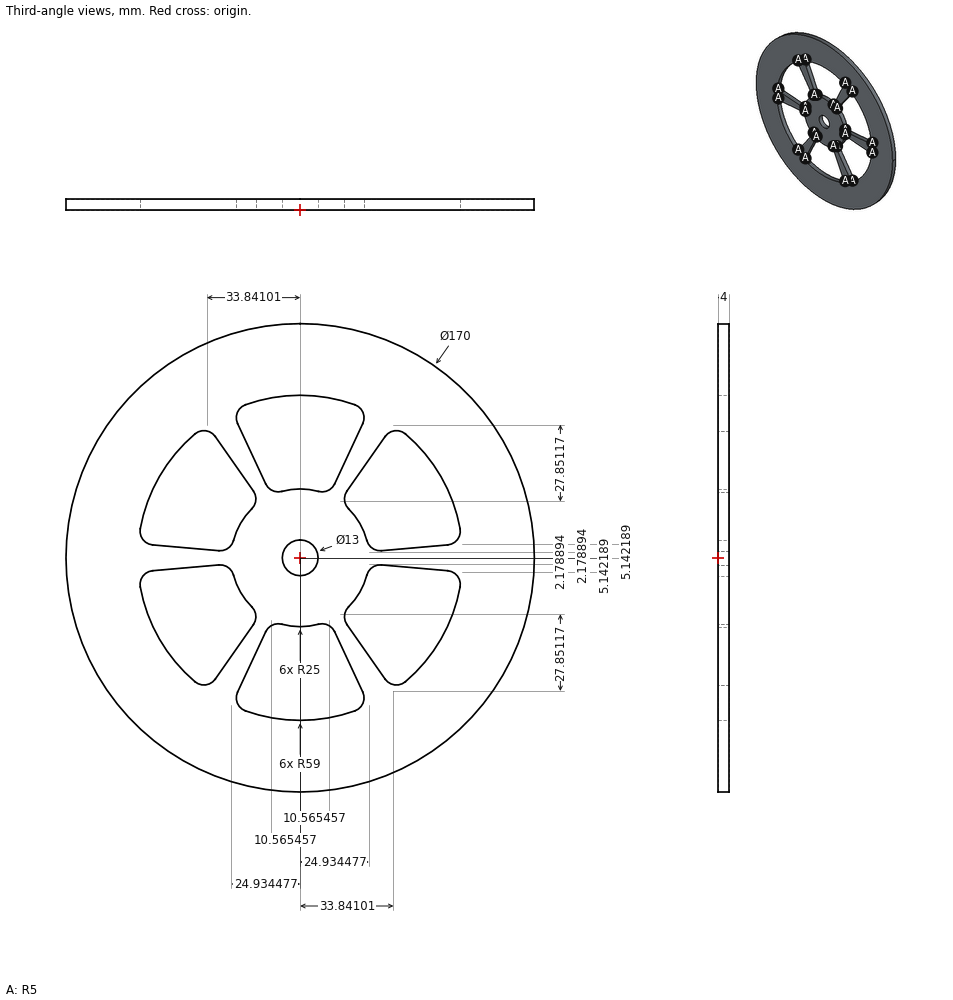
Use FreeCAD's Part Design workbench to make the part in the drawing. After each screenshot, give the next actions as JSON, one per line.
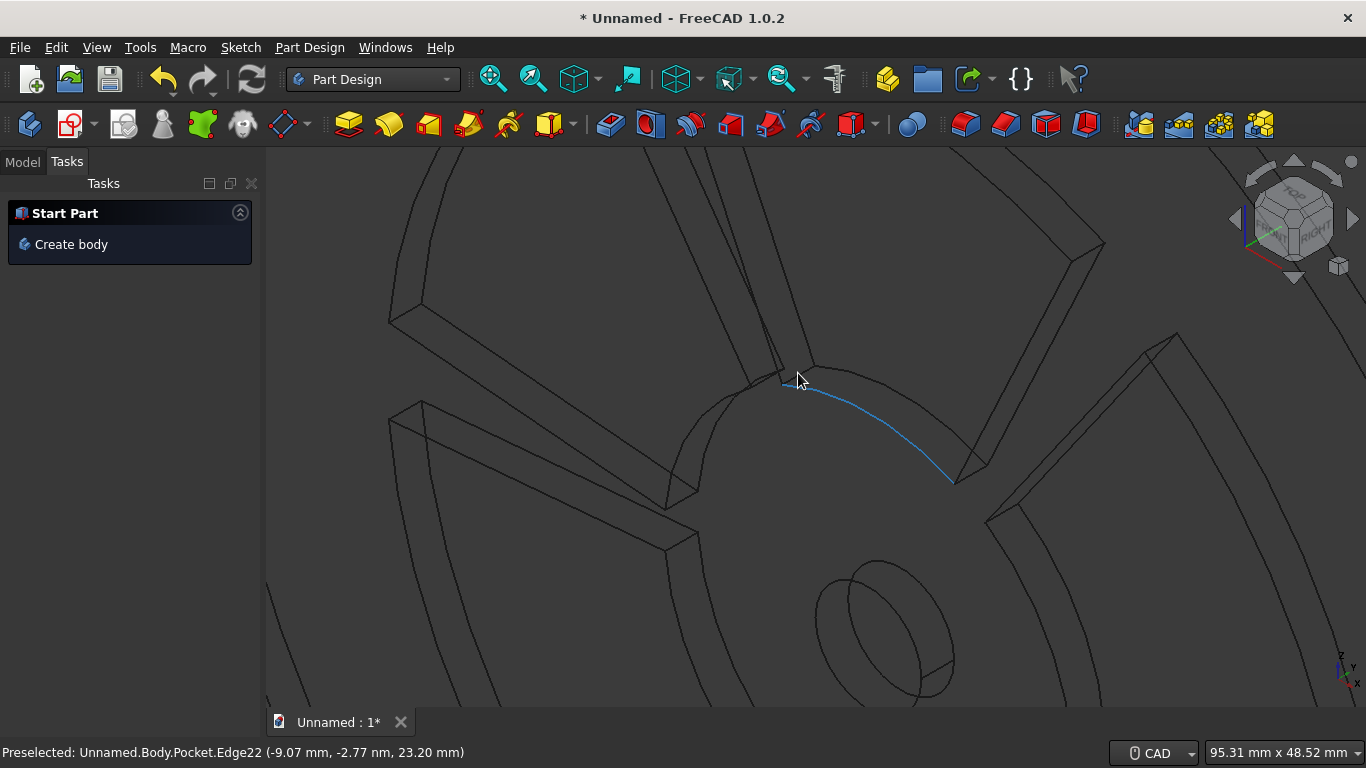
{"action": "left_click", "coordinate": [799, 374]}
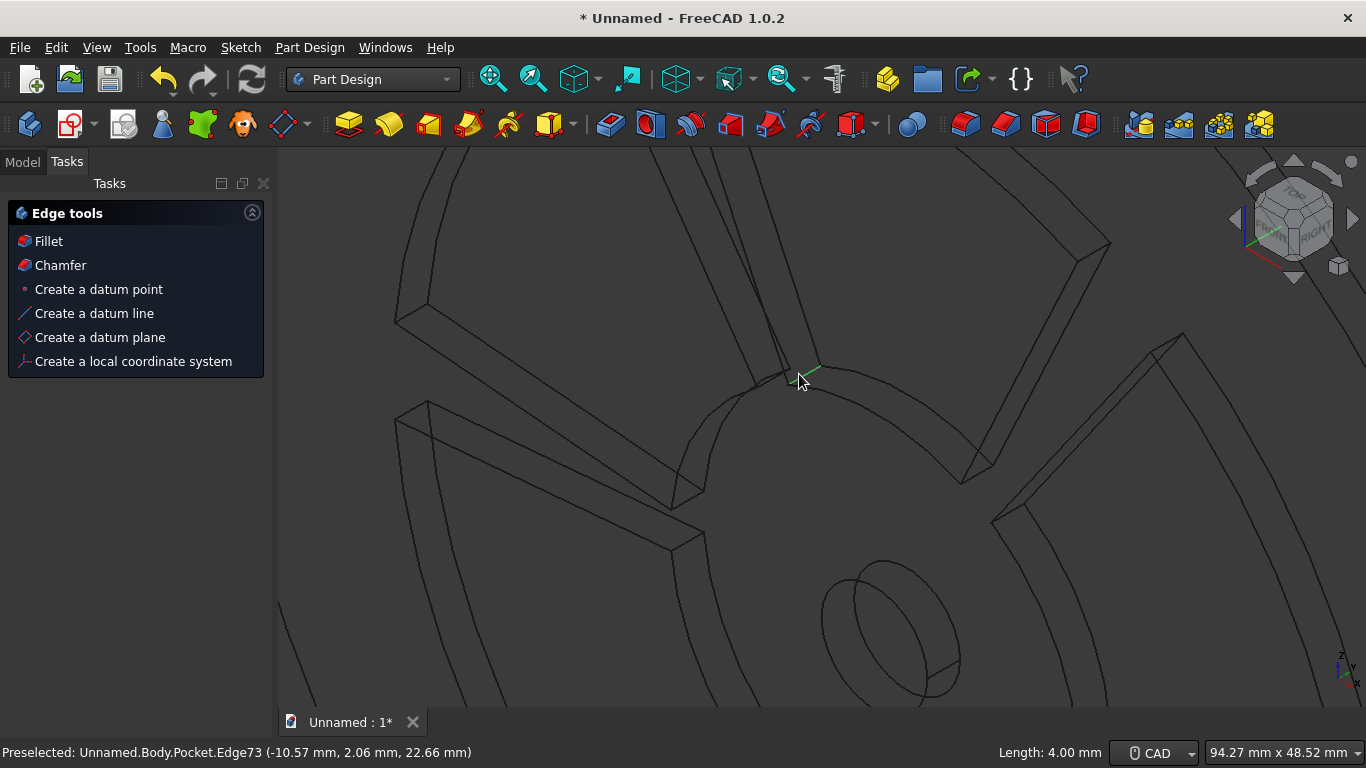
{"action": "left_click", "coordinate": [977, 474], "text": "ctrl"}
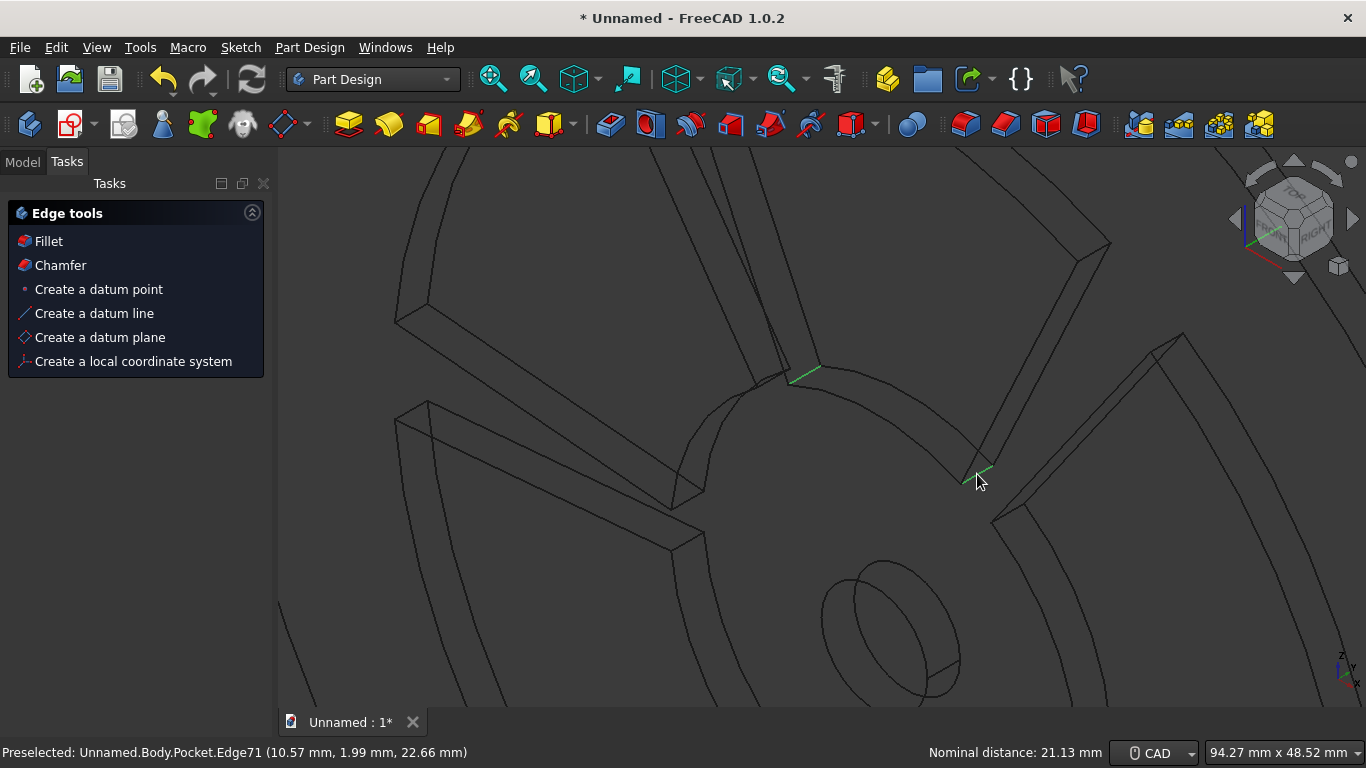
{"action": "left_click", "coordinate": [1094, 251], "text": "ctrl"}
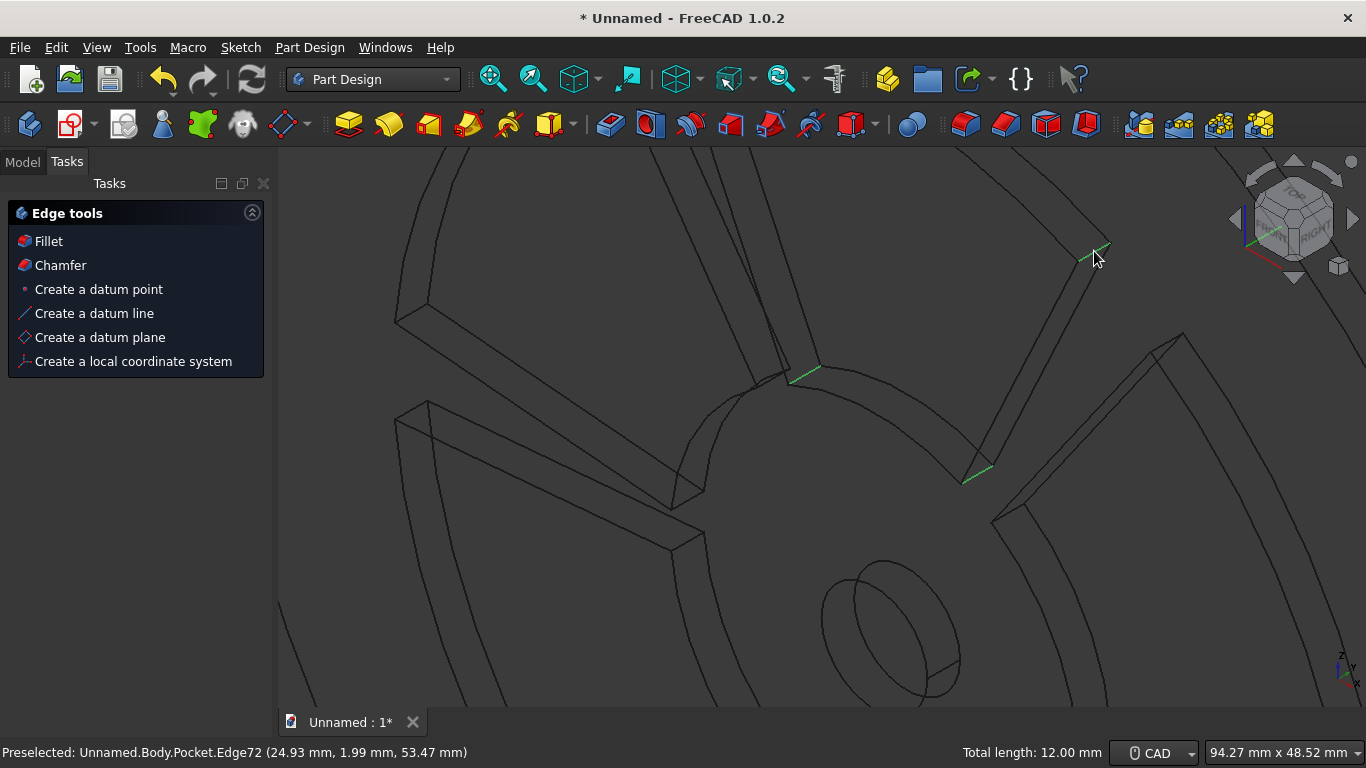
{"action": "left_click", "coordinate": [688, 500], "text": "ctrl"}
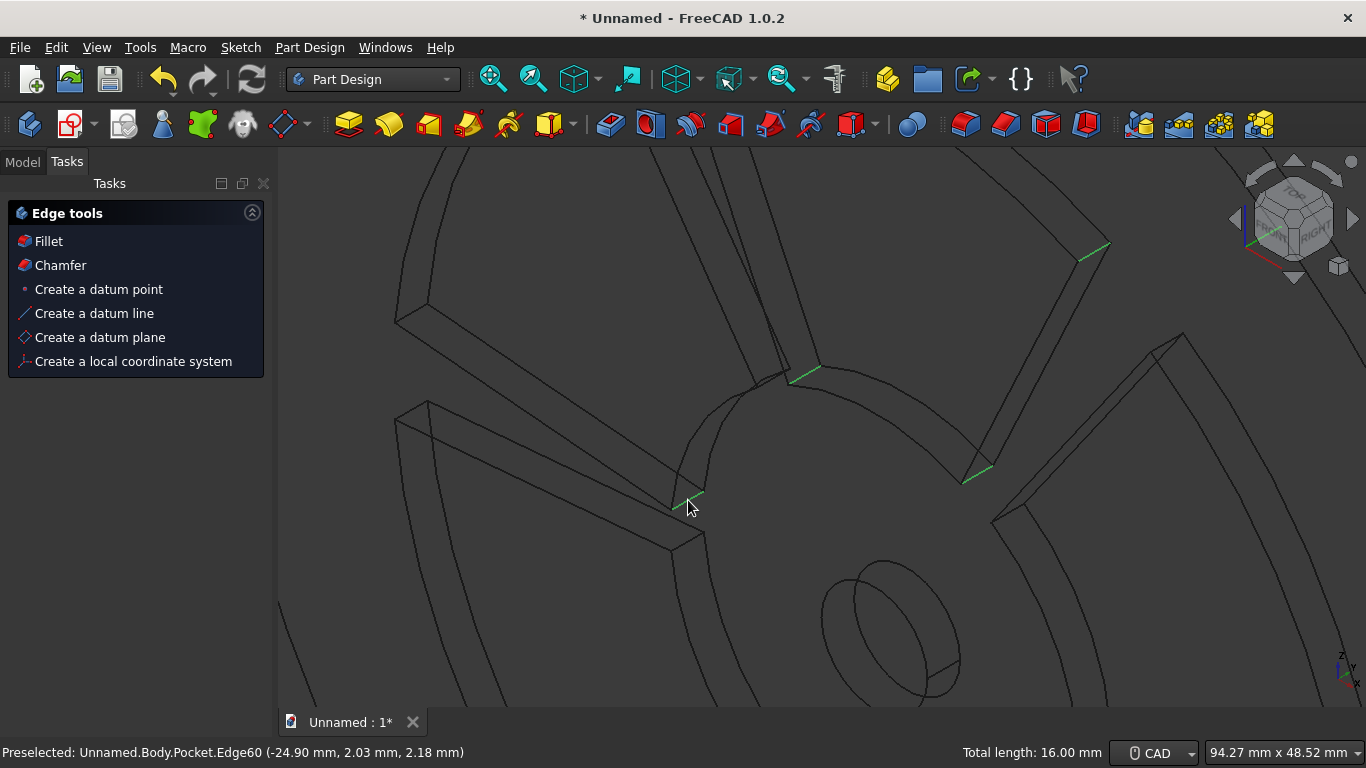
{"action": "left_click", "coordinate": [774, 377], "text": "ctrl"}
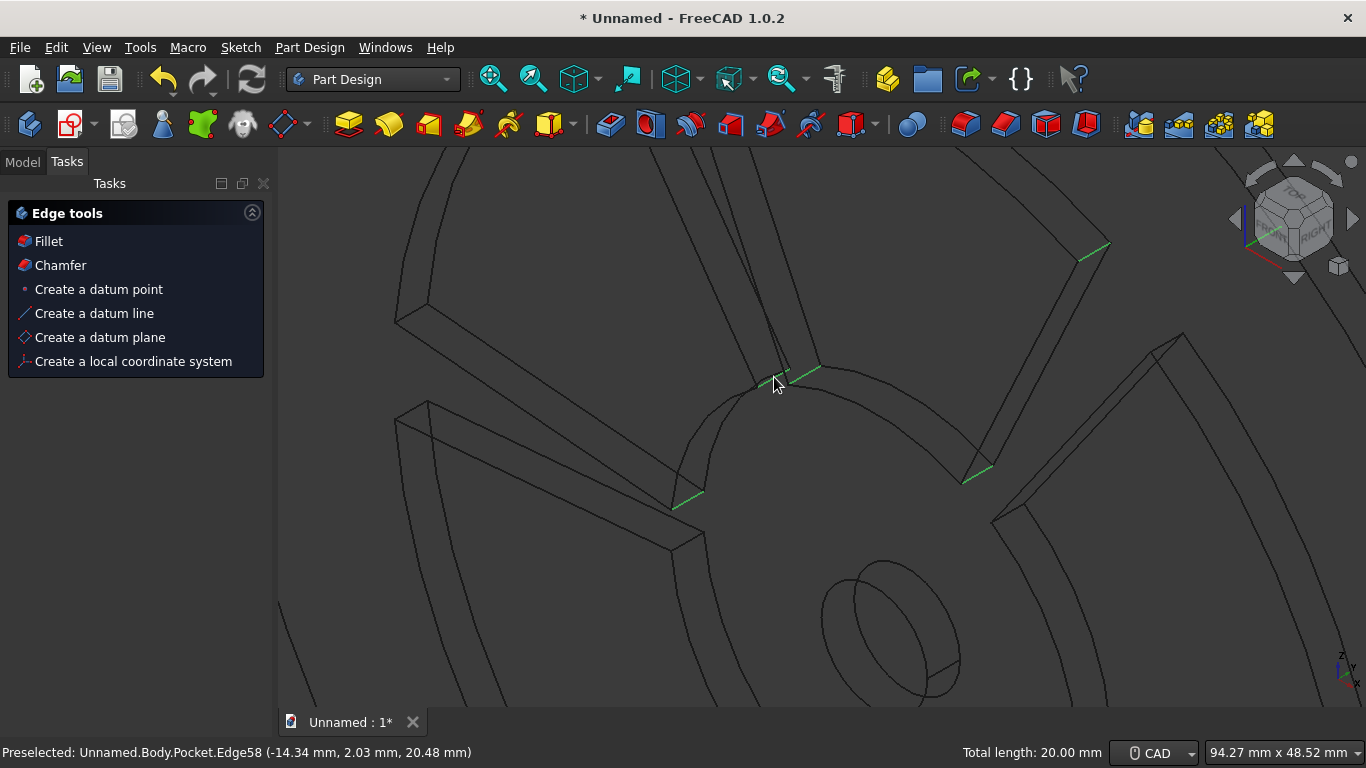
{"action": "left_click", "coordinate": [411, 312], "text": "ctrl"}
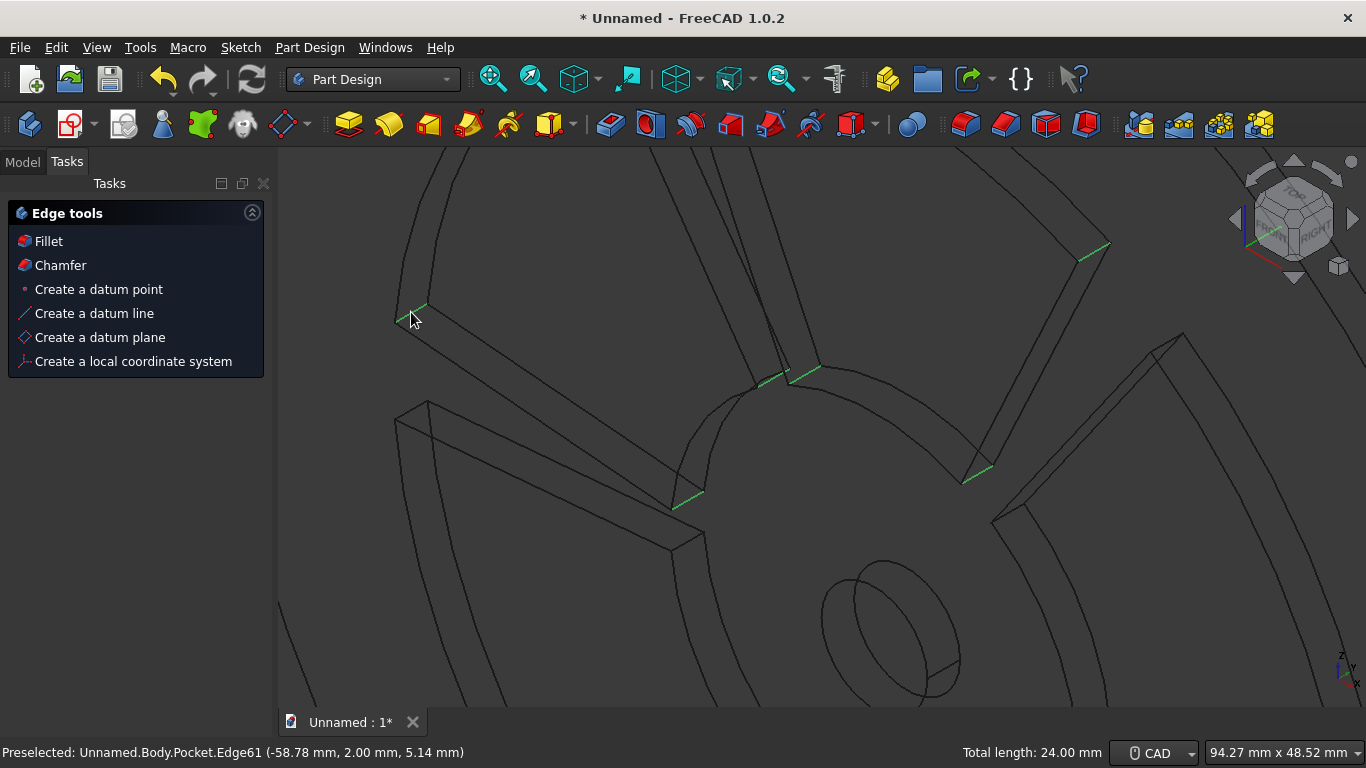
{"action": "left_click", "coordinate": [1014, 508], "text": "ctrl"}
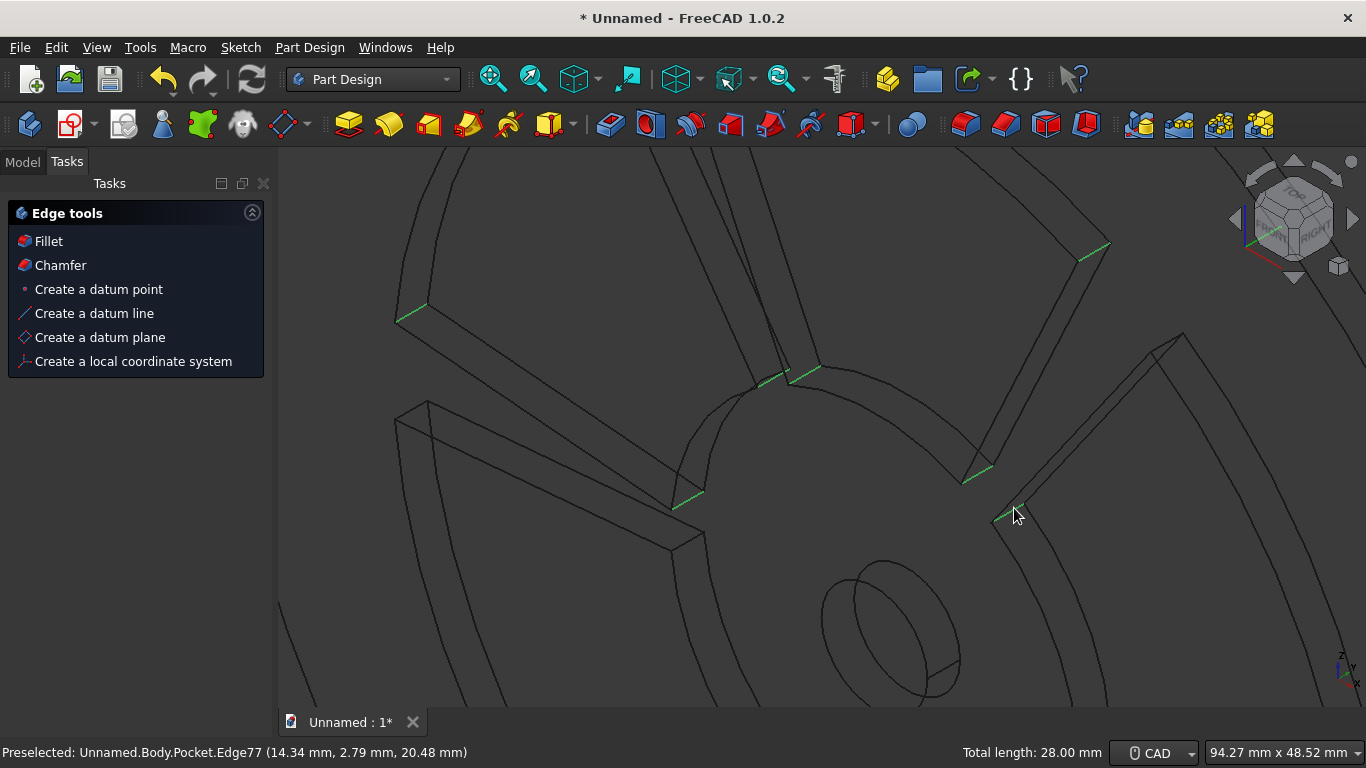
{"action": "left_click", "coordinate": [1167, 342], "text": "ctrl"}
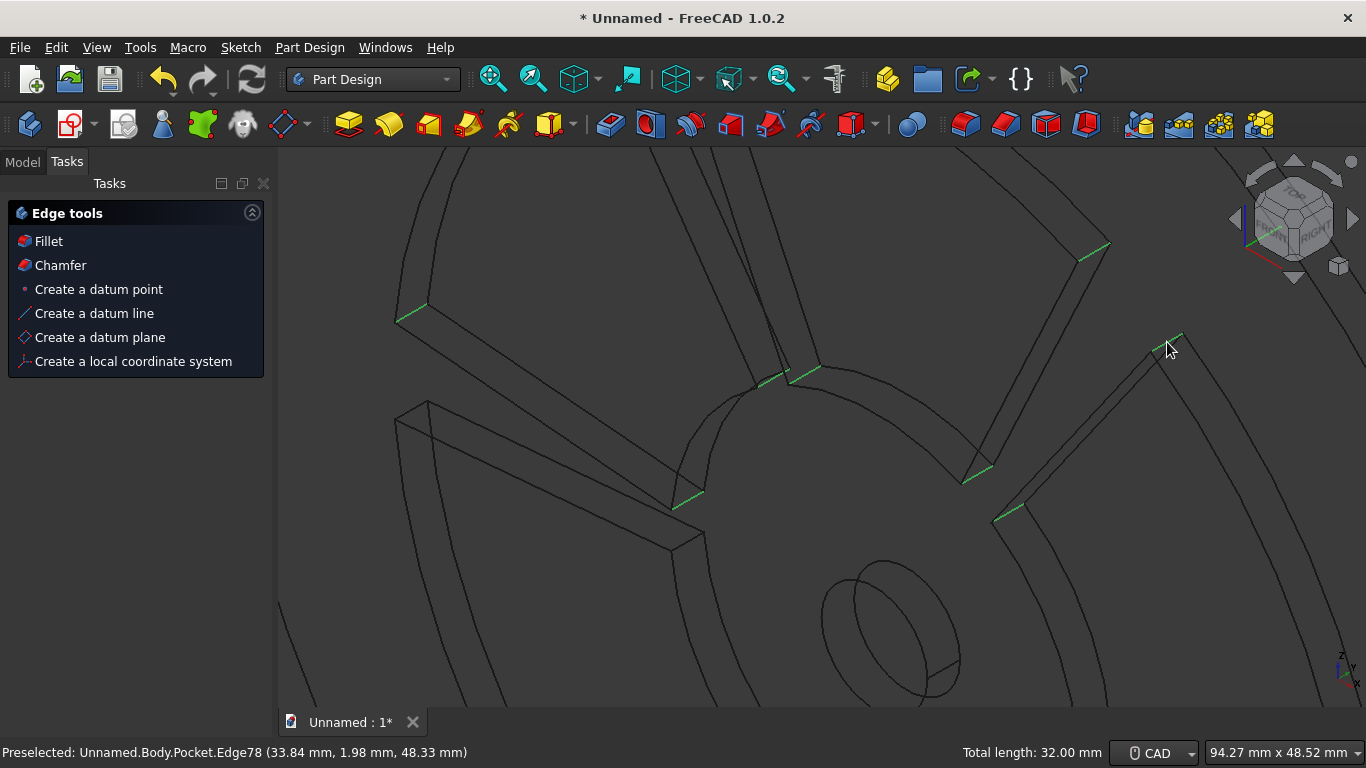
{"action": "left_click", "coordinate": [688, 541], "text": "ctrl"}